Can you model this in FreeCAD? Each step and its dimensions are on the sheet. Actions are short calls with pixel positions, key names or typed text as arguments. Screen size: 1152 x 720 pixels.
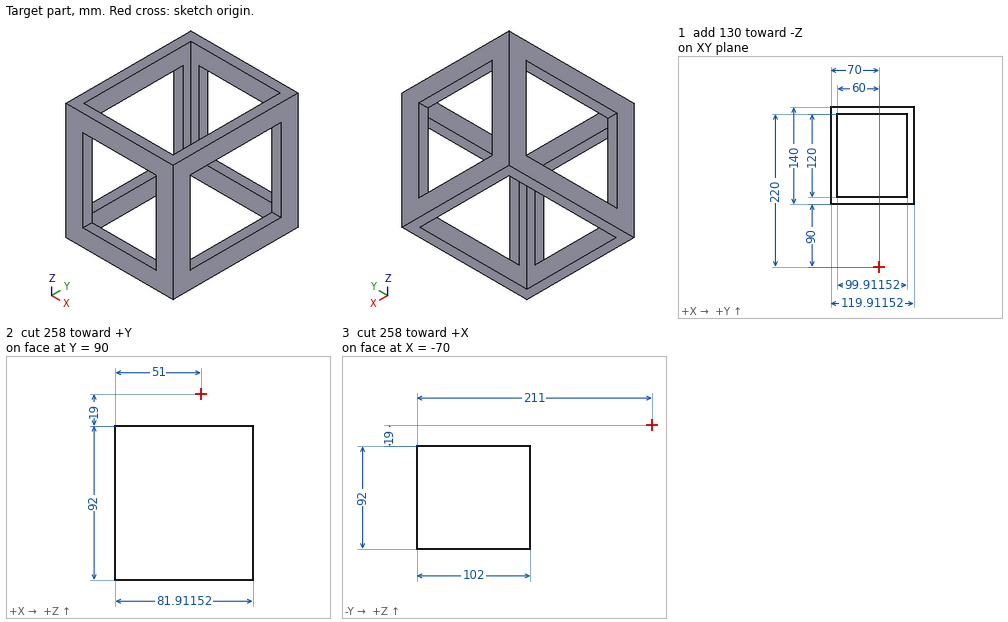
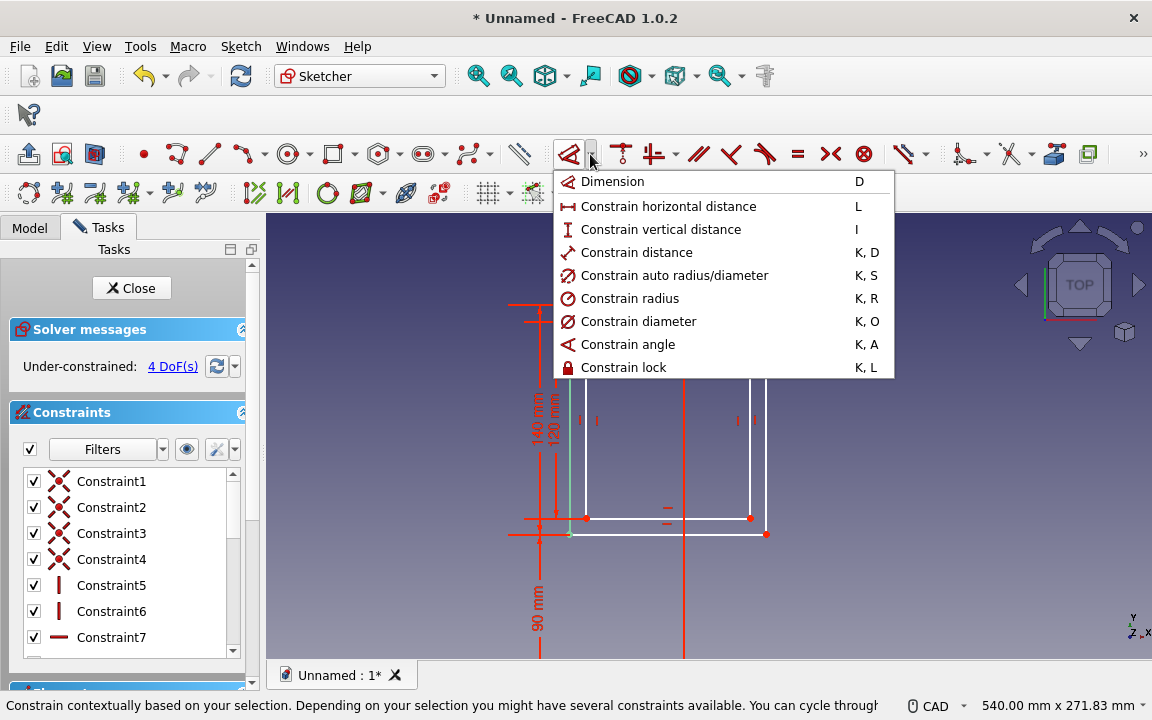
click(724, 206)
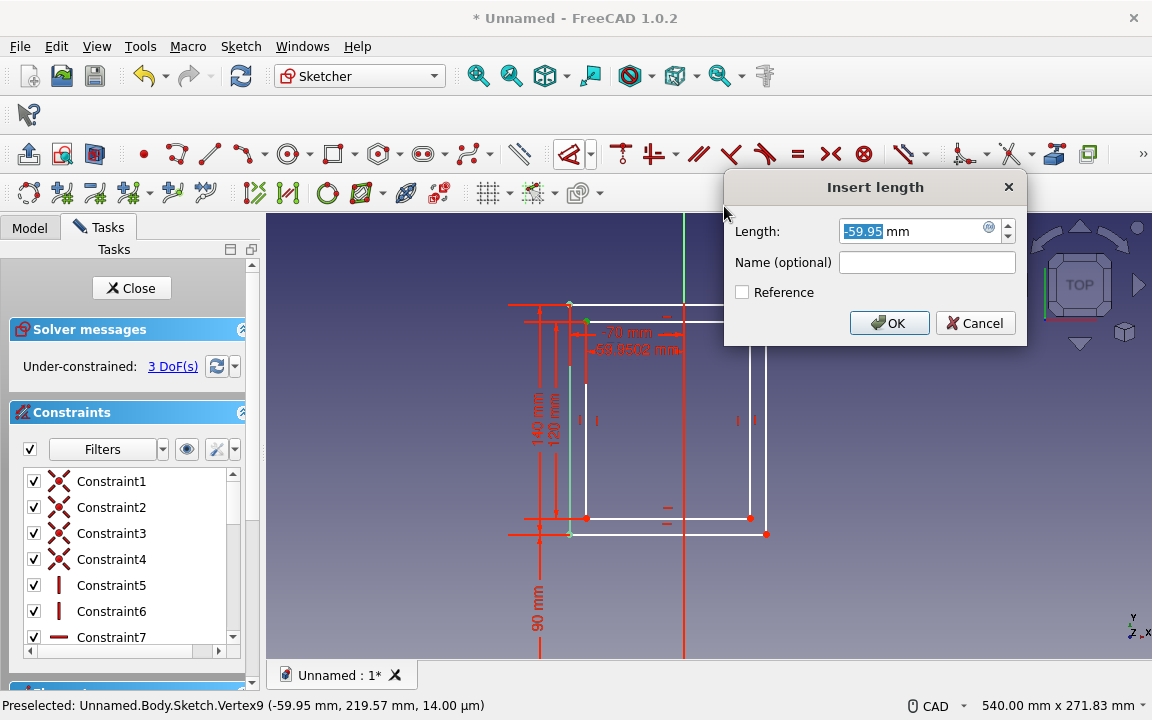
text(-60)
key(Return)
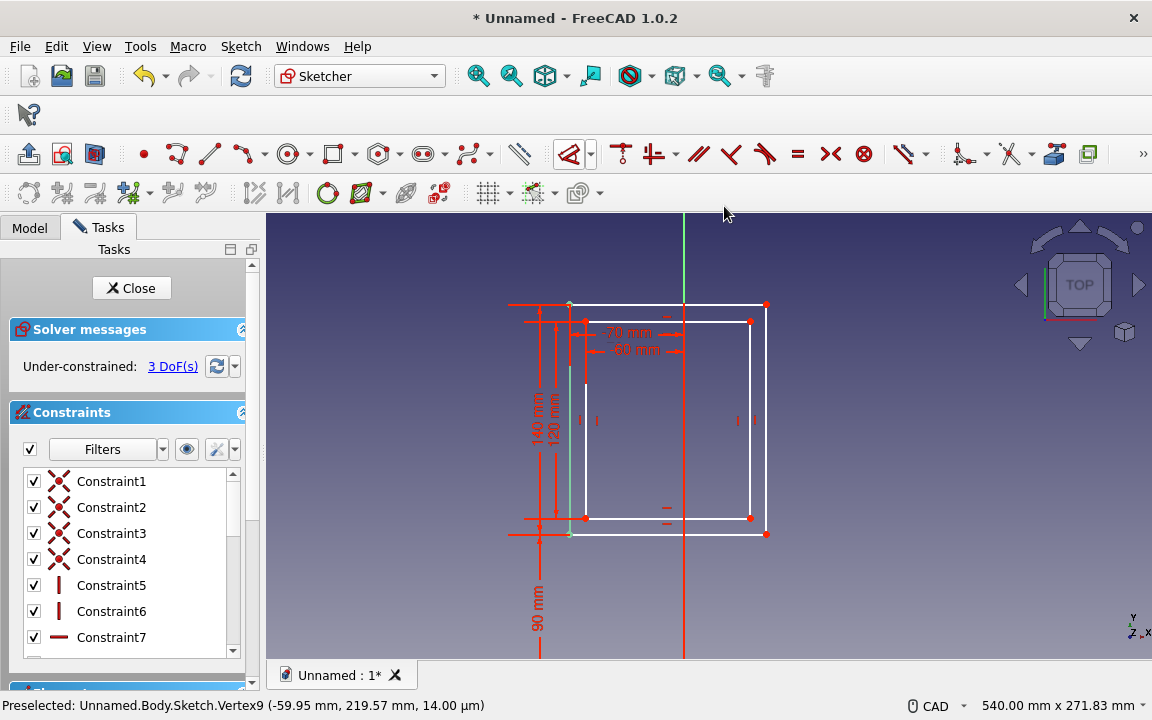
click(586, 322)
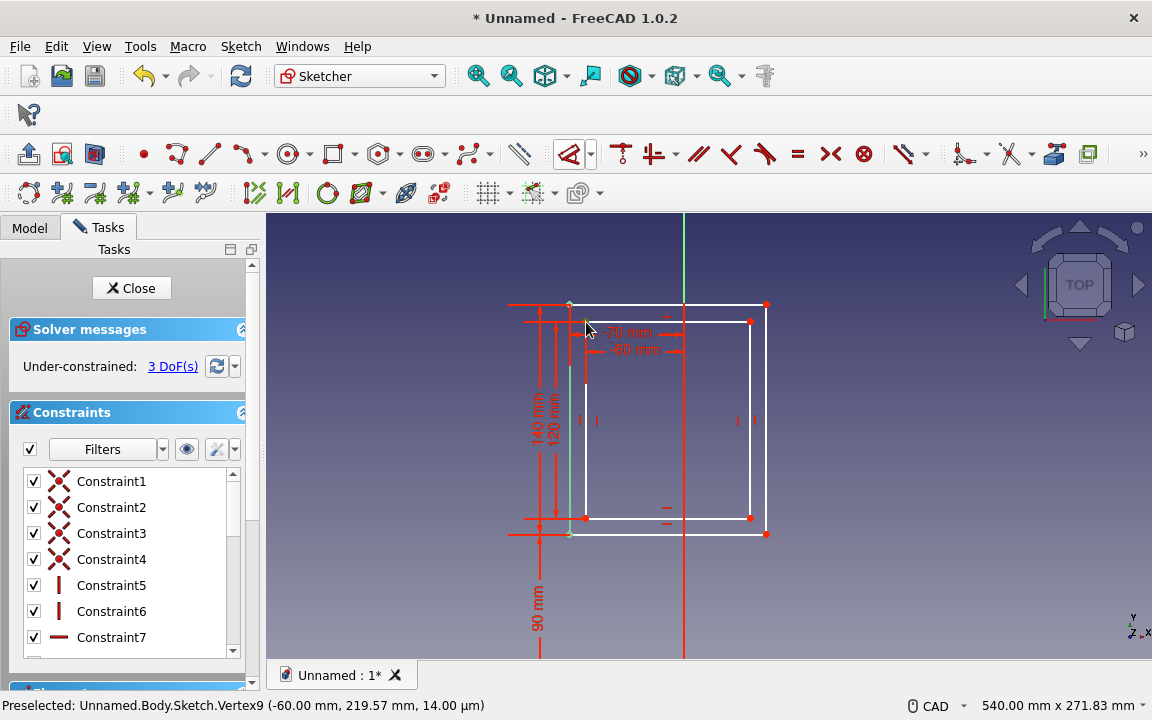
key(i)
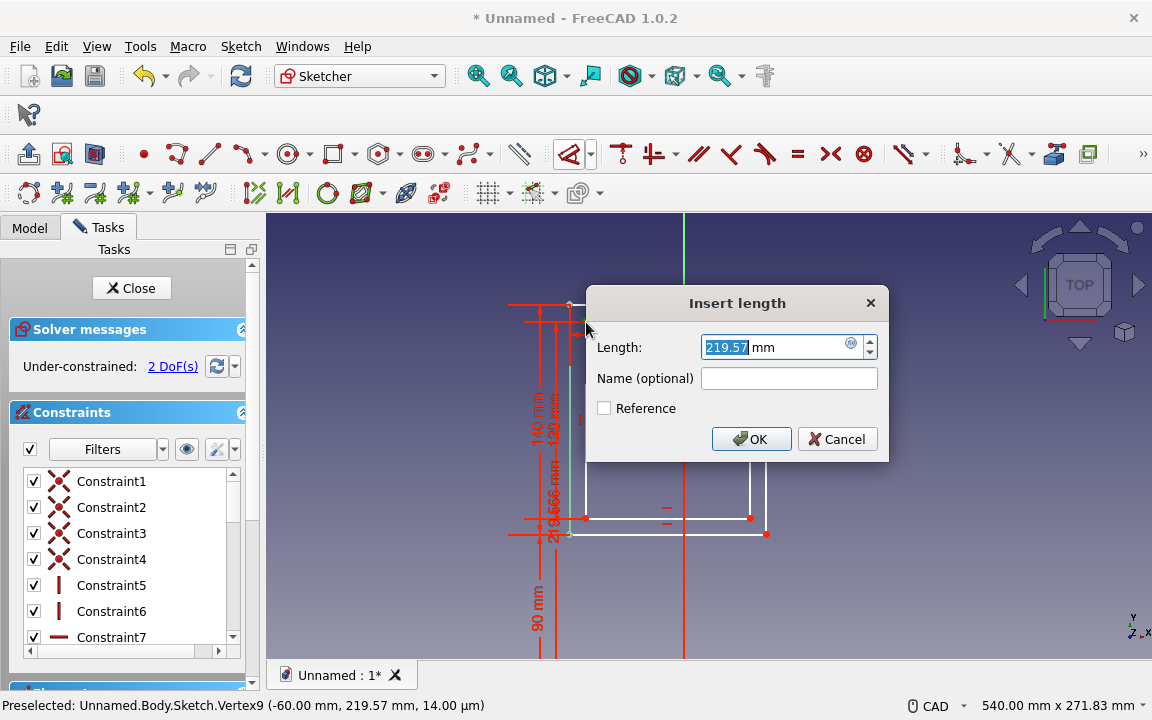
text(220)
key(Return)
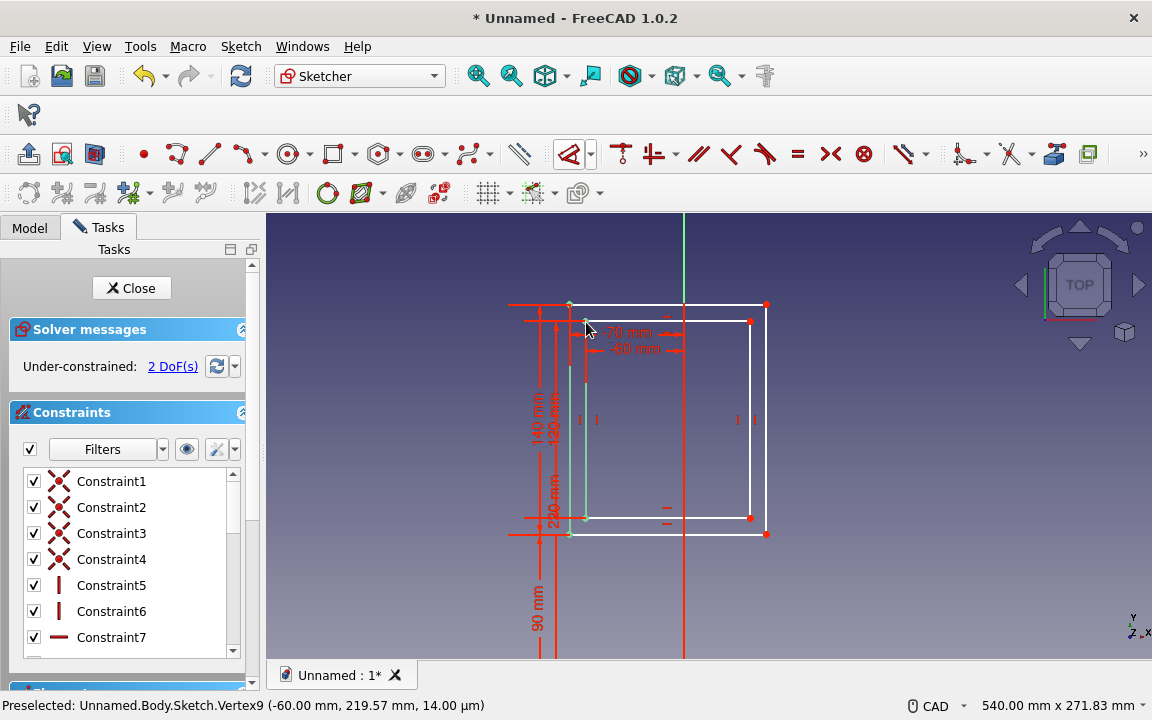
click(635, 518)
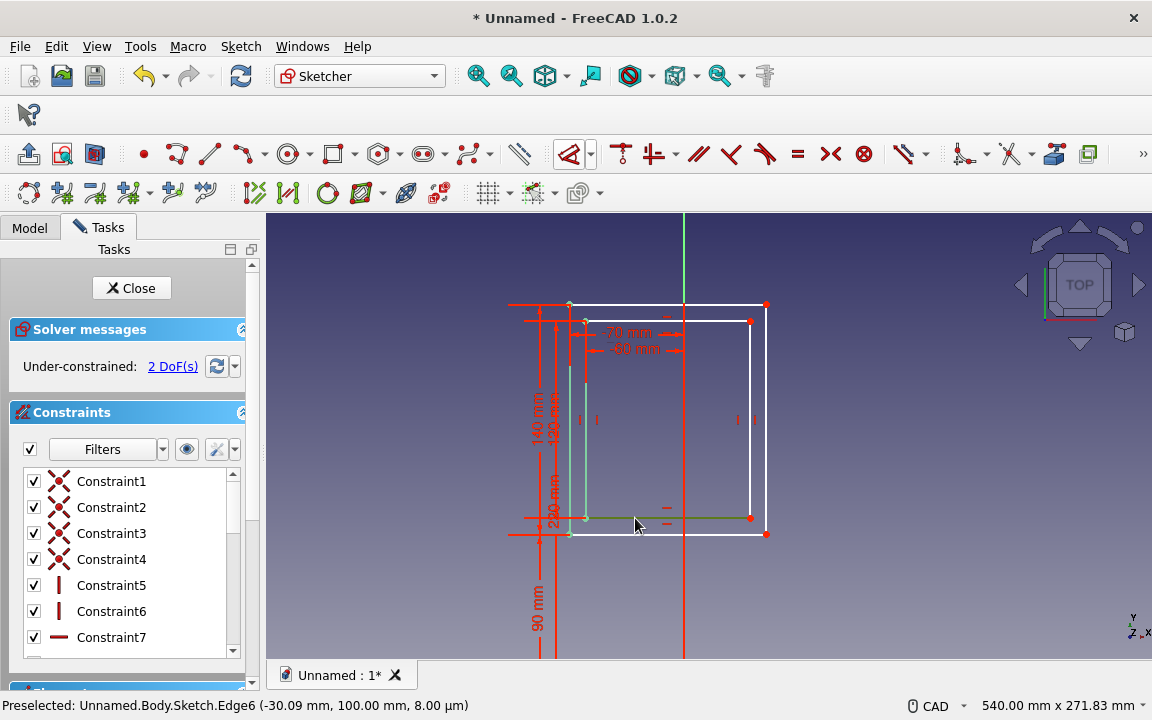
click(590, 154)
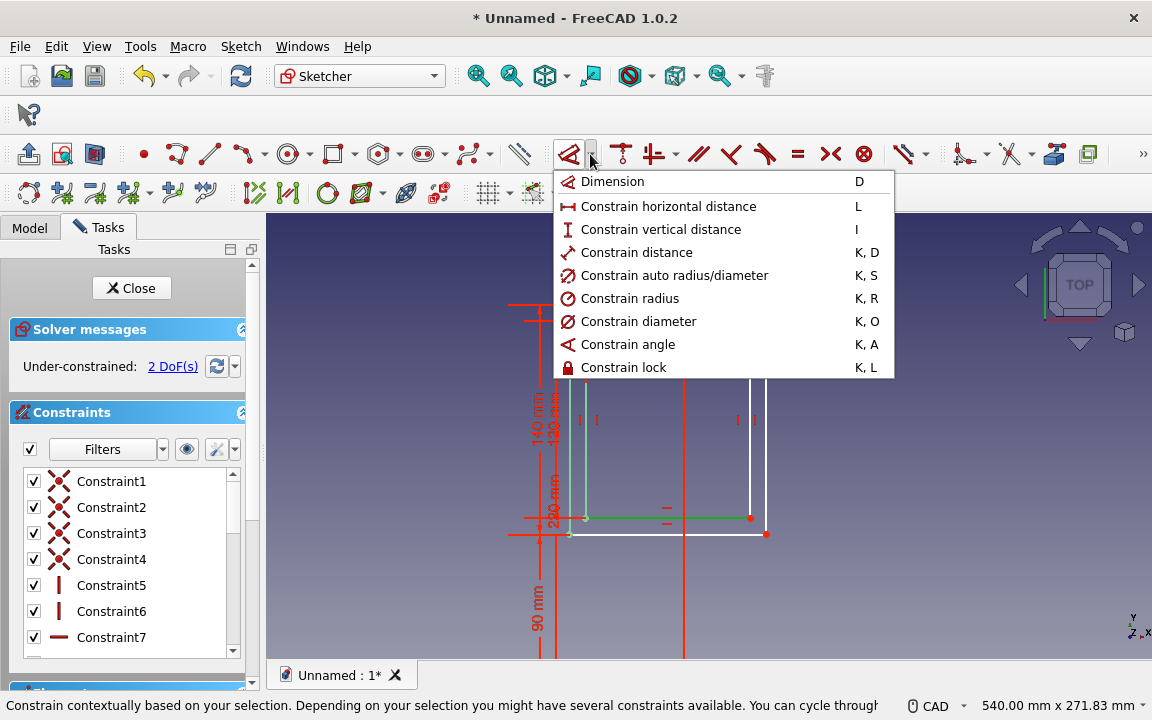
click(724, 206)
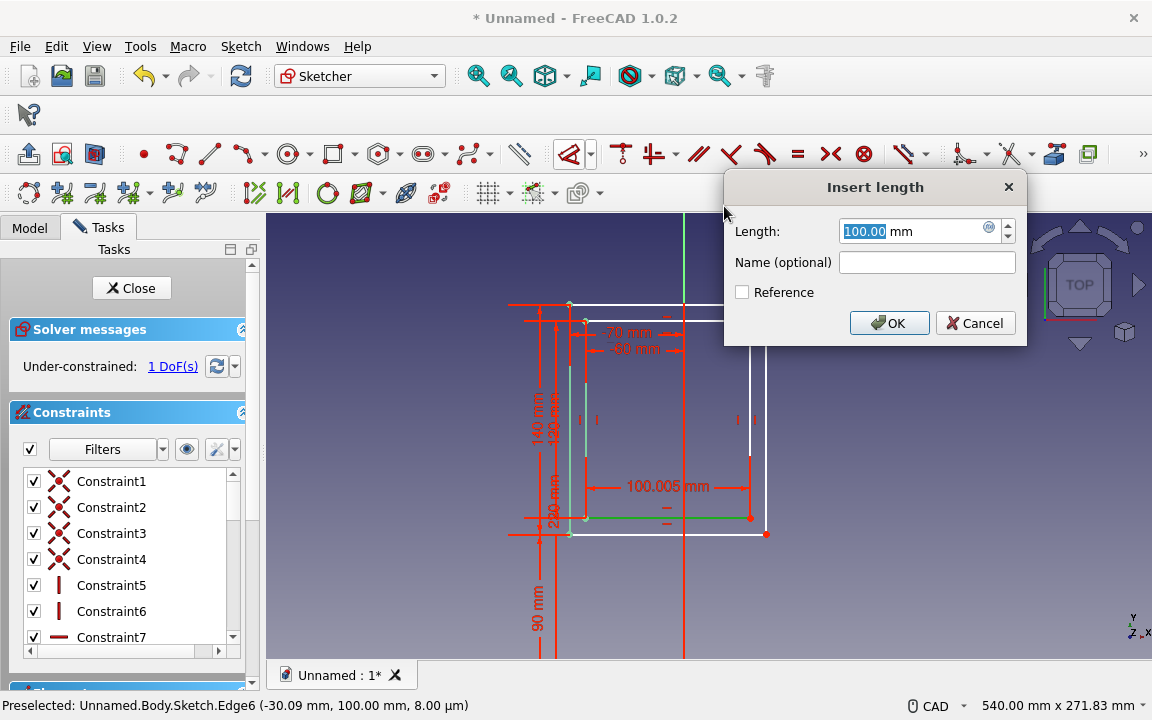
text(99.91152)
key(Return)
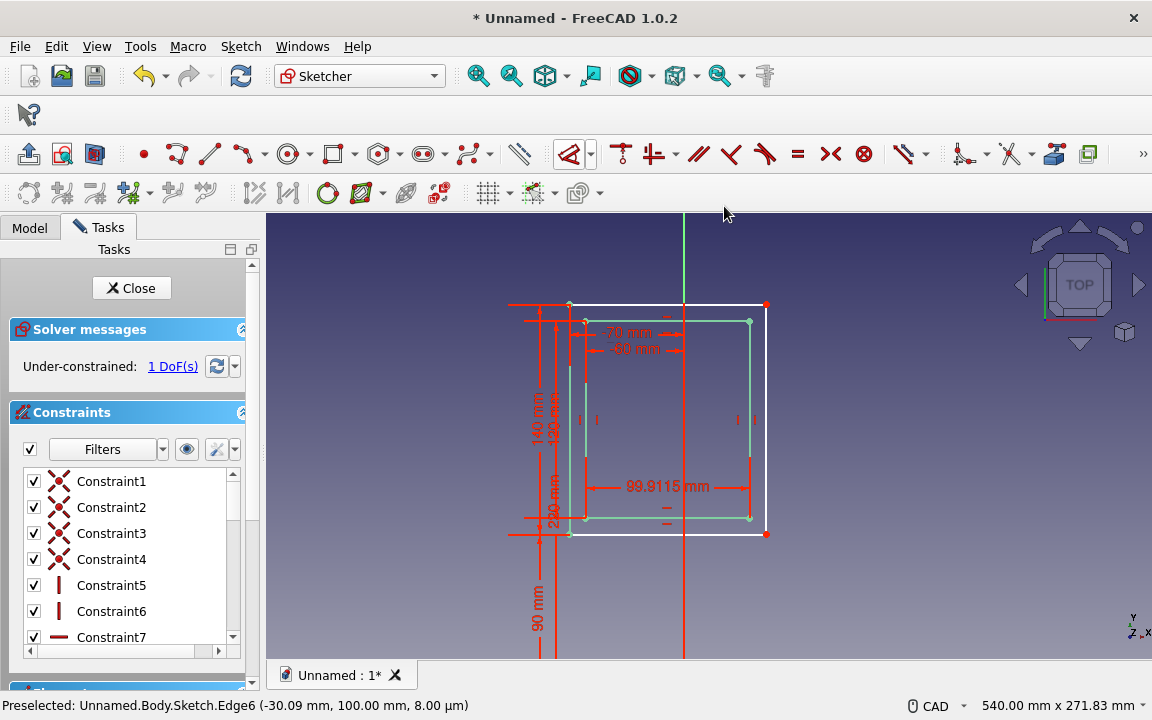
click(629, 535)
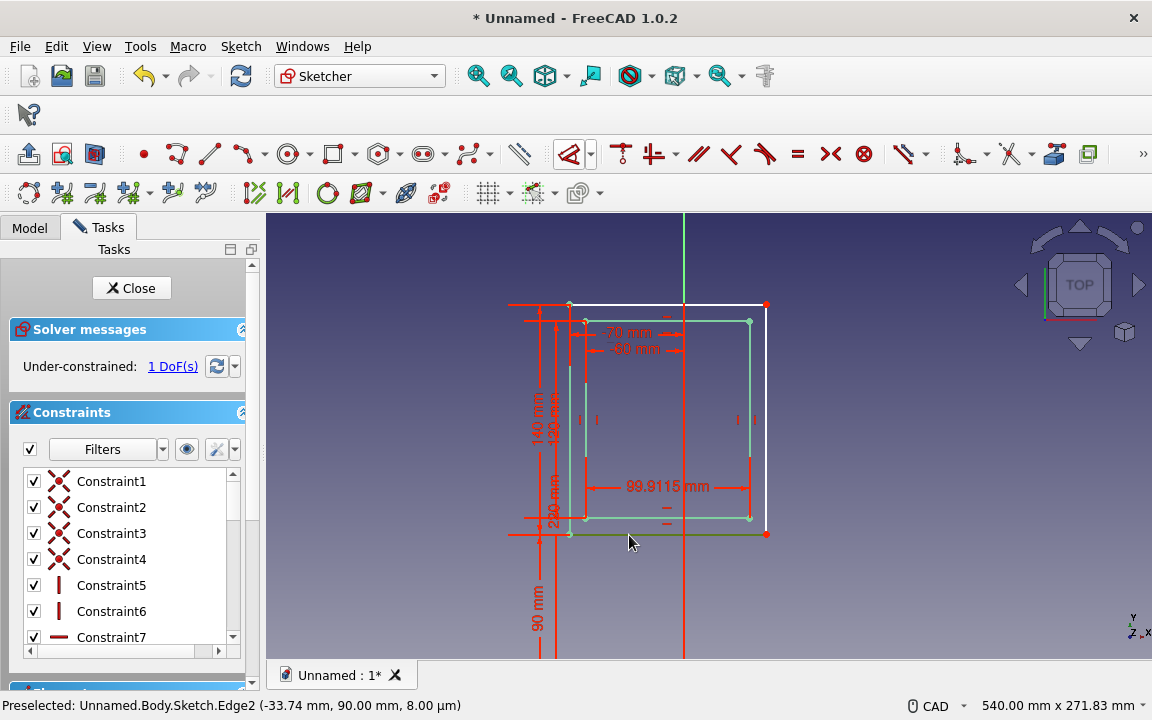
key(l)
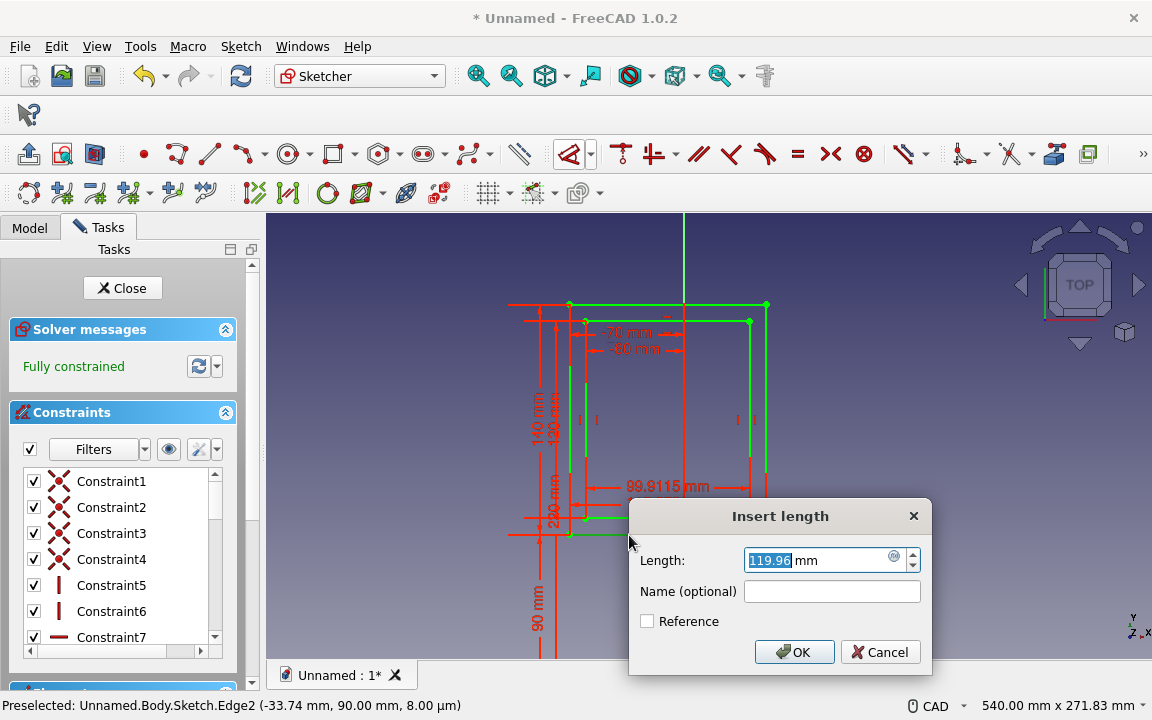
text(119.91152)
key(Return)